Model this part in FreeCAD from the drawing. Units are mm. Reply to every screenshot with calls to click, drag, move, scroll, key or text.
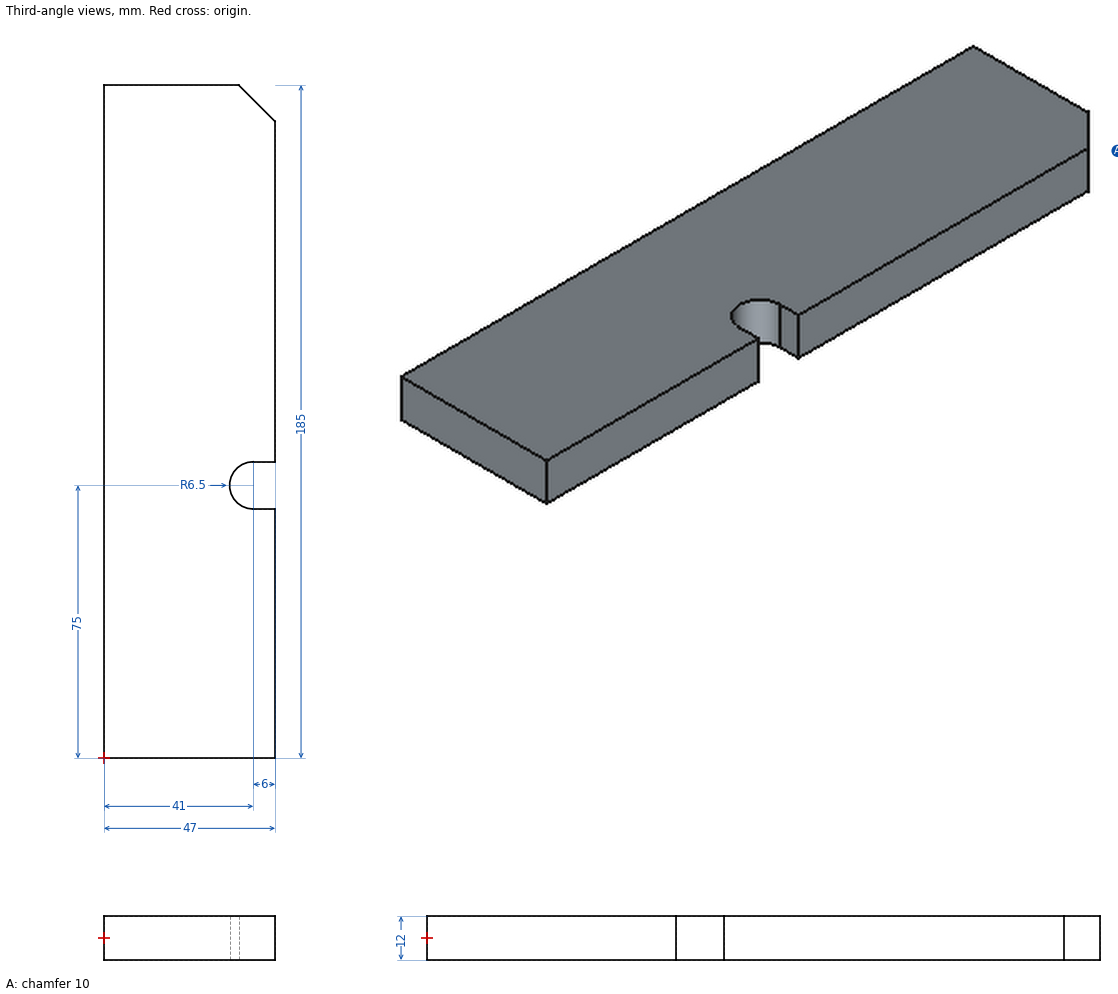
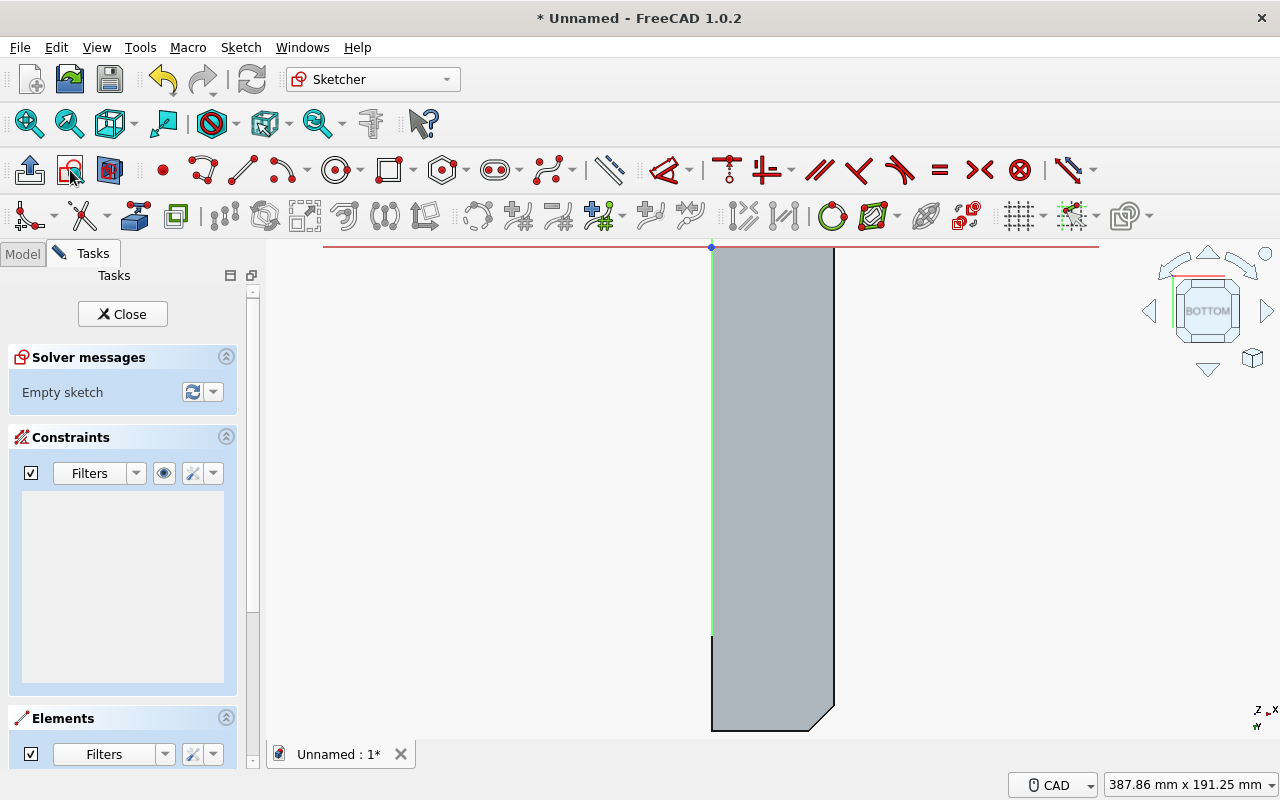
scroll(832, 438, up, 11)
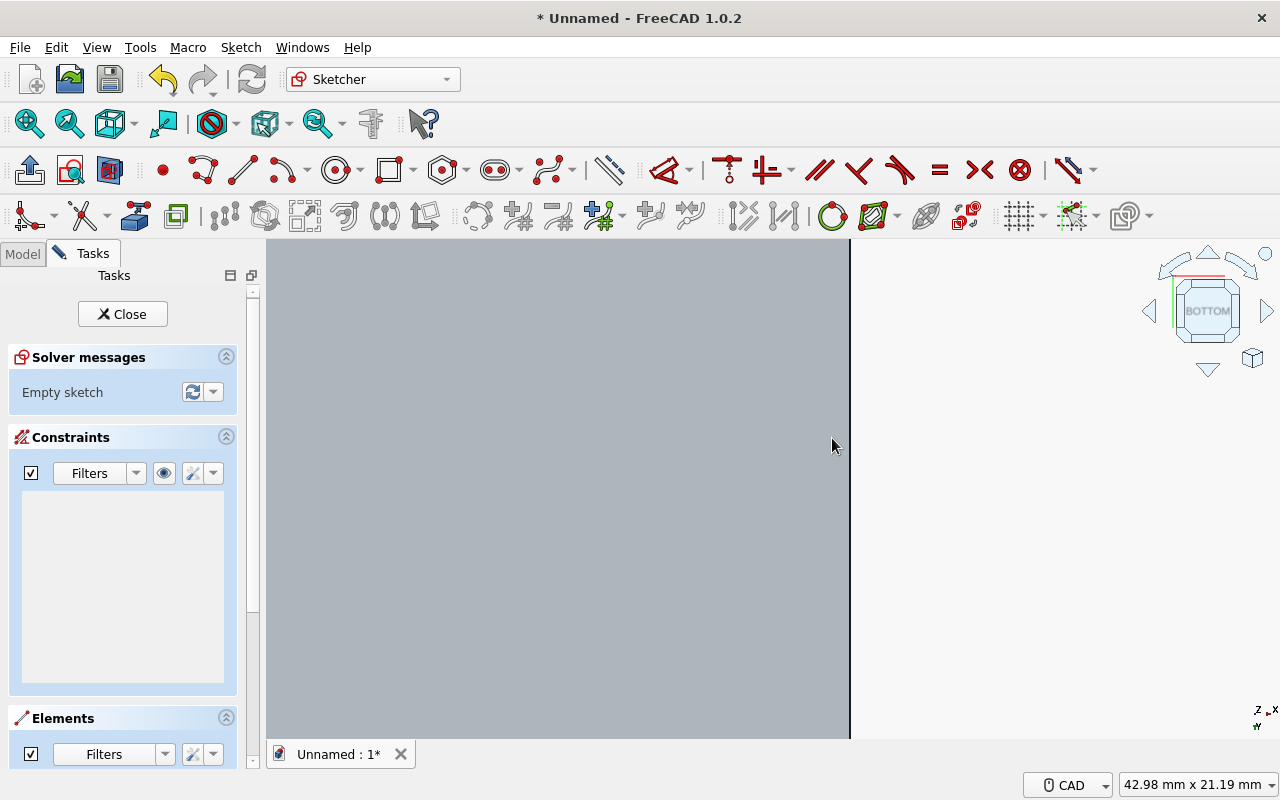
click(204, 170)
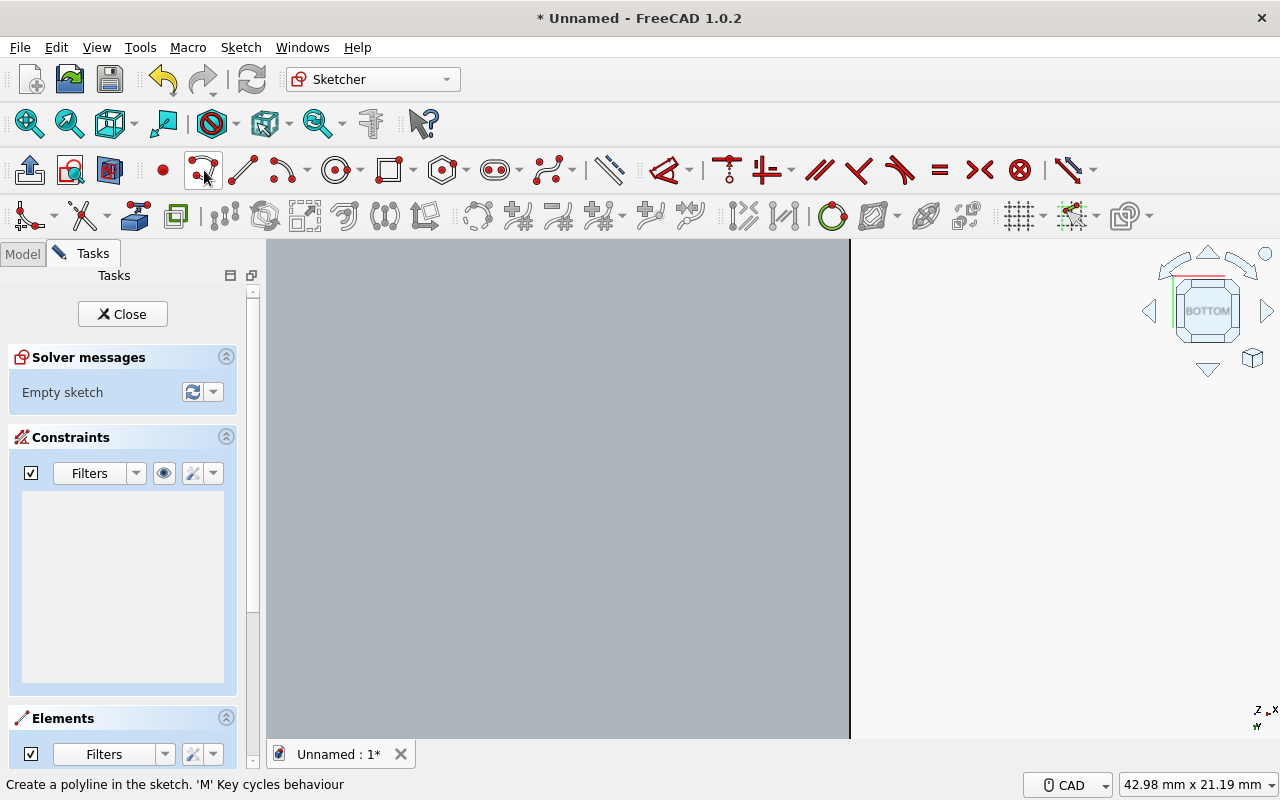
click(708, 636)
click(850, 636)
click(850, 329)
click(708, 329)
right_click(708, 329)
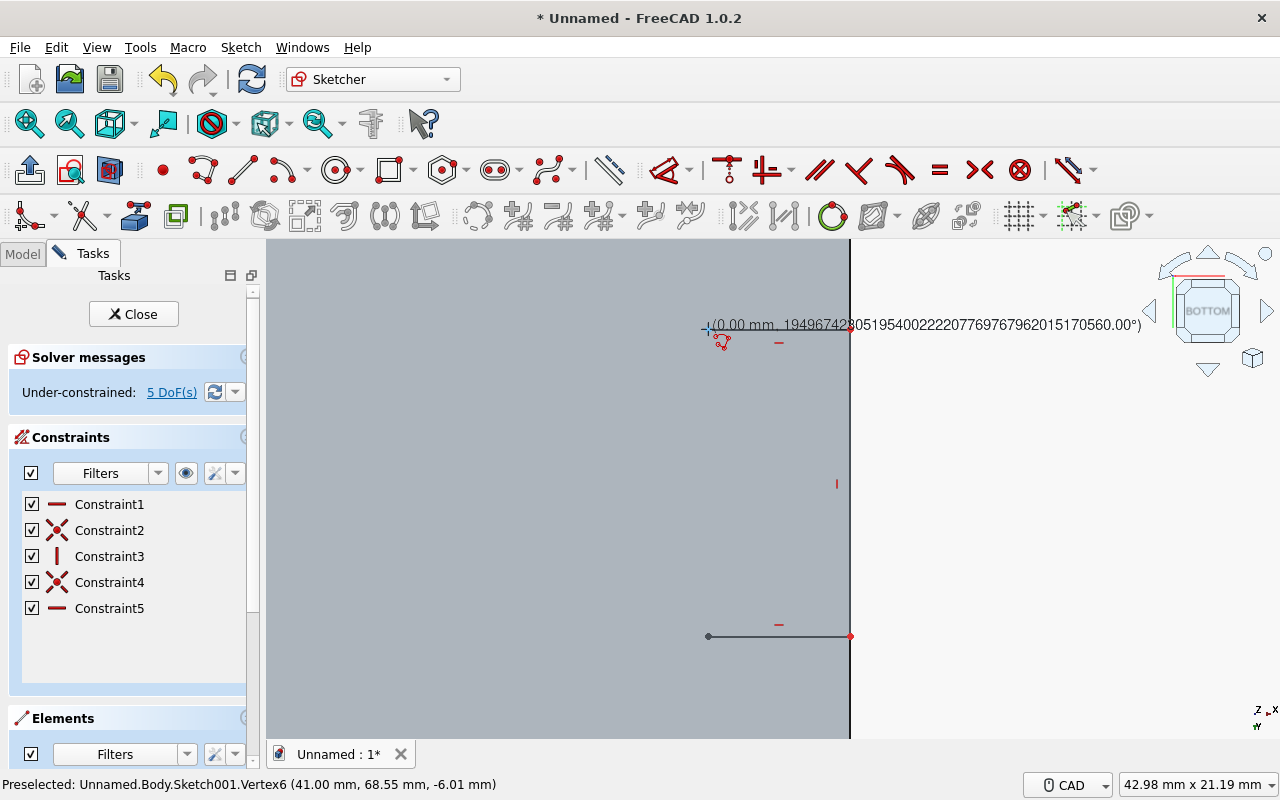
key(g)
key(3)
key(a)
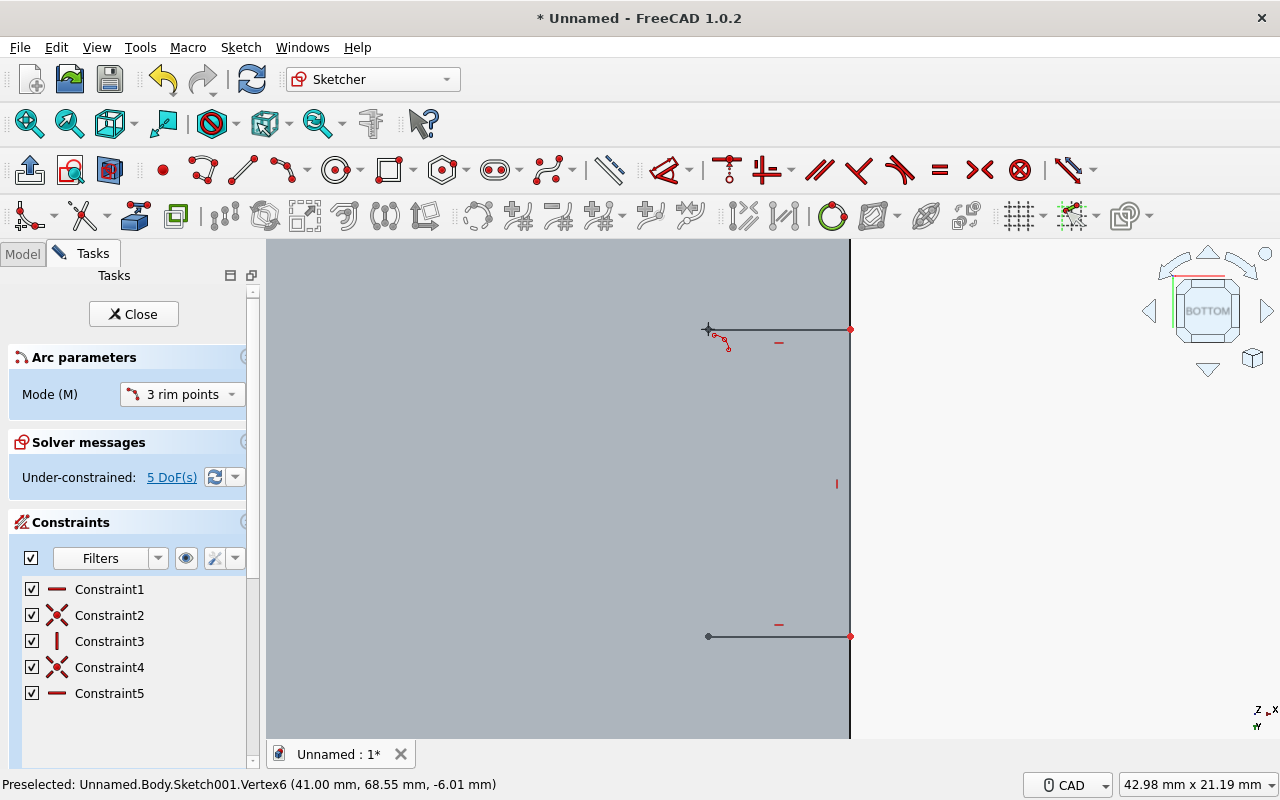
click(708, 330)
click(708, 637)
click(555, 482)
key(Escape)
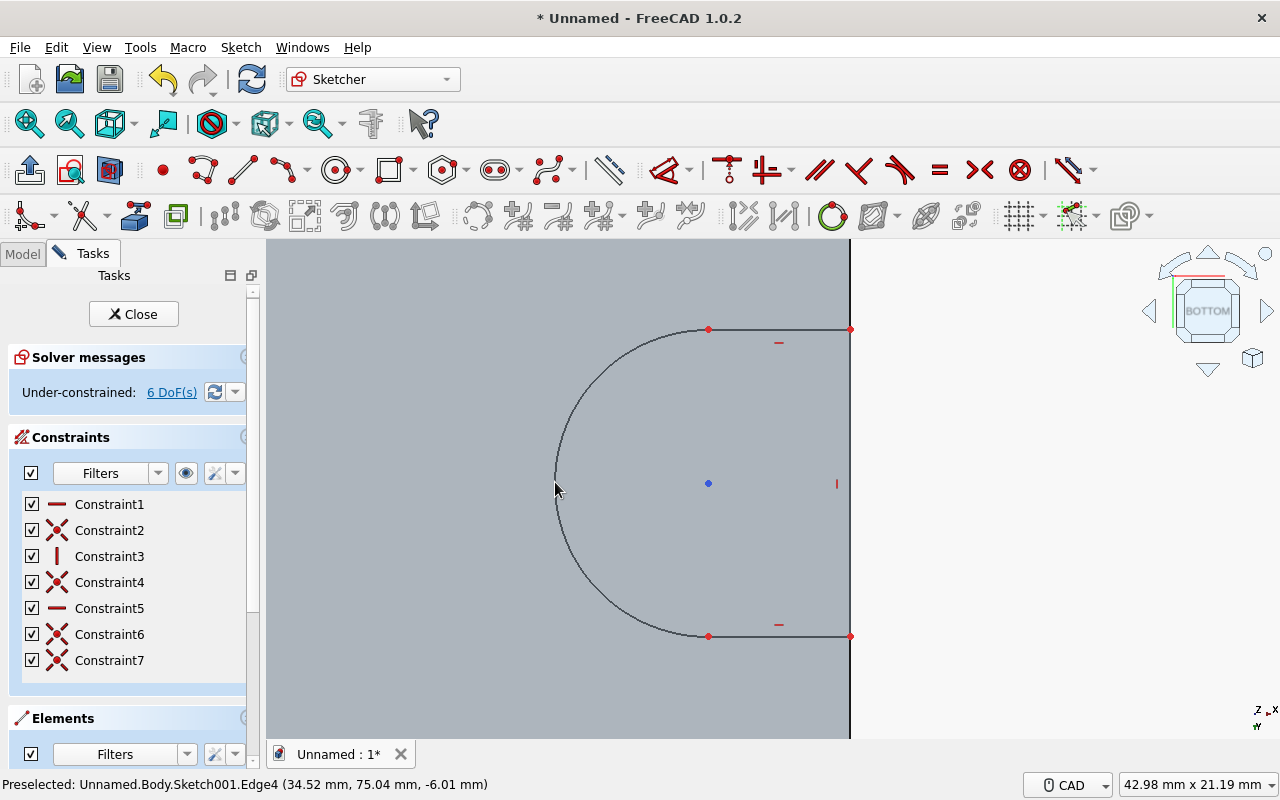
click(751, 637)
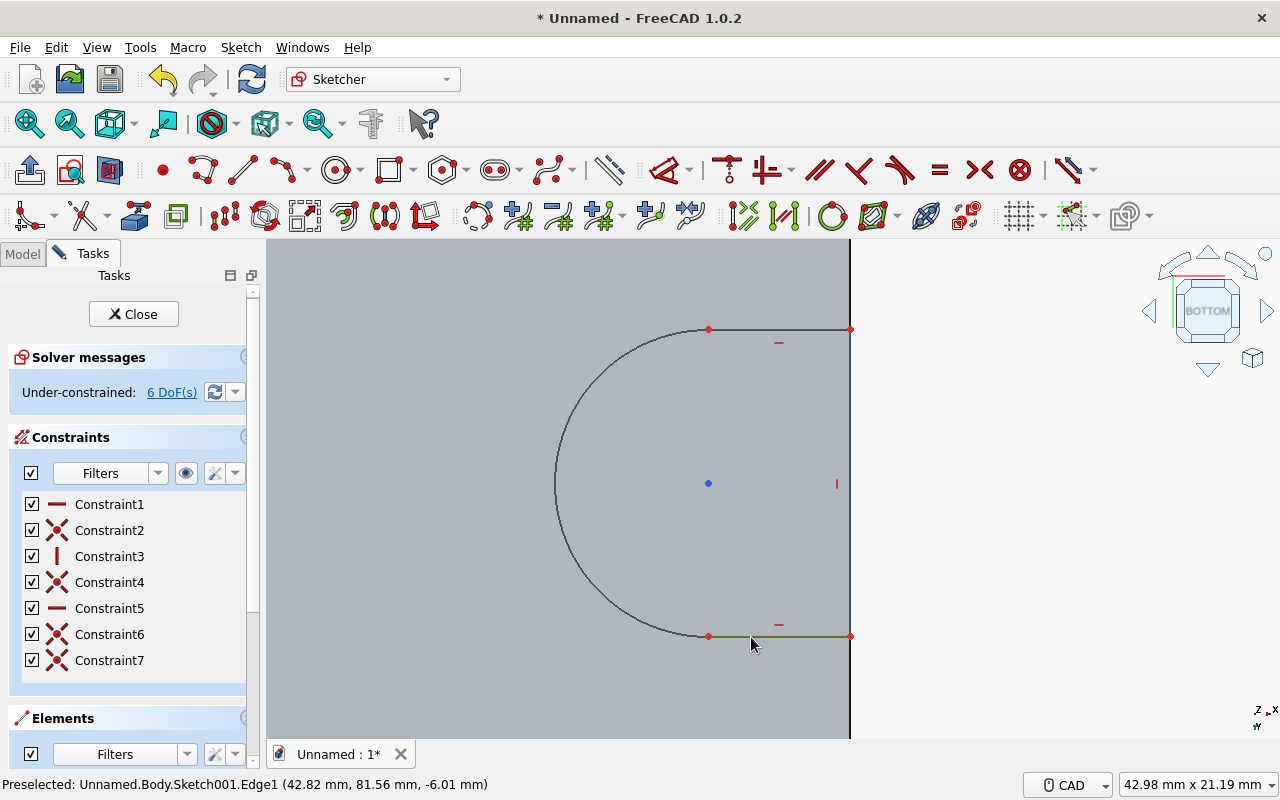
click(584, 393)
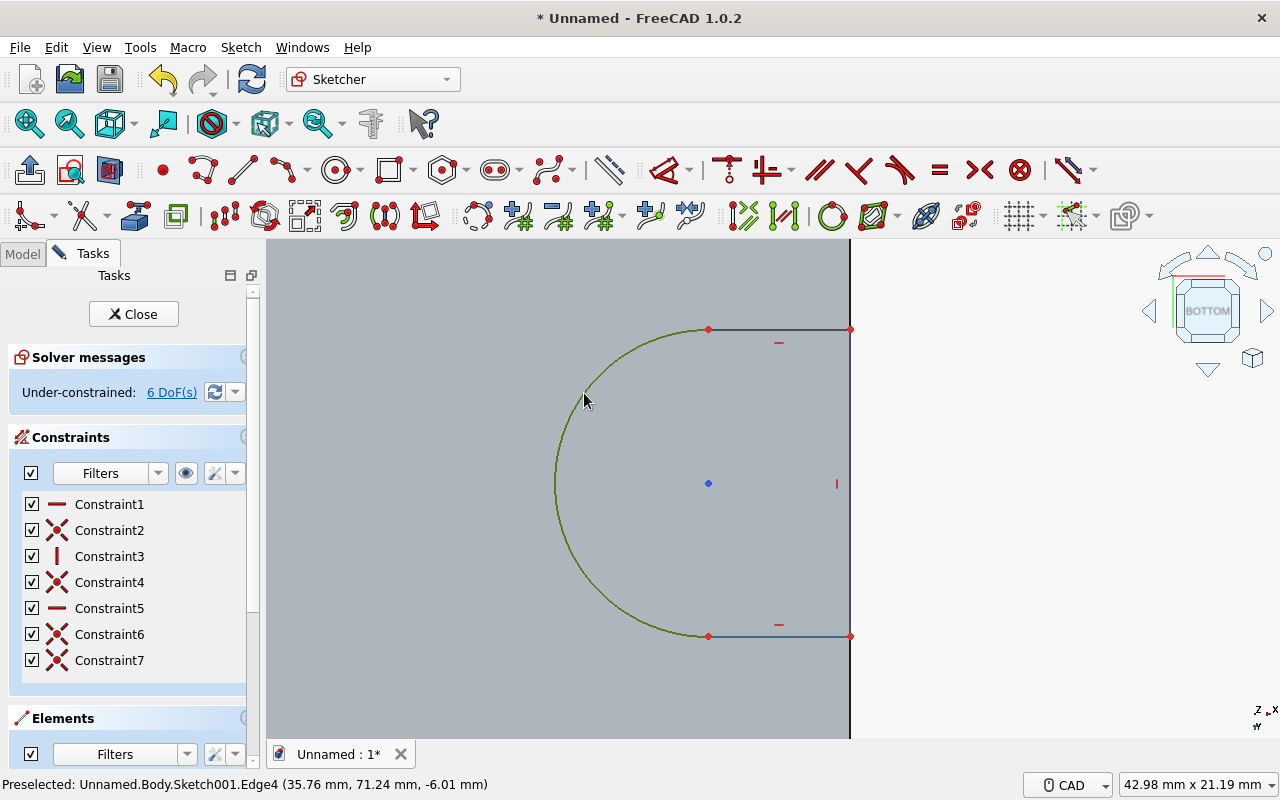
click(900, 170)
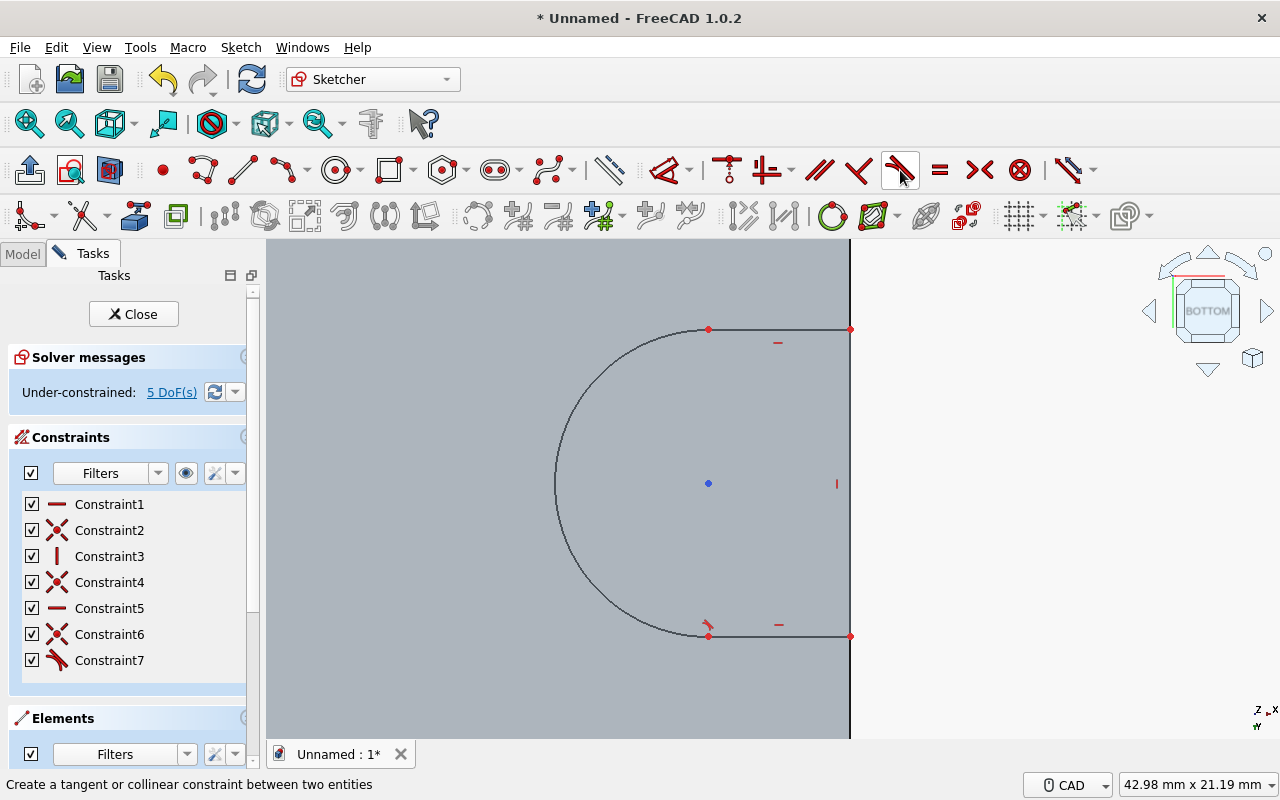
click(807, 330)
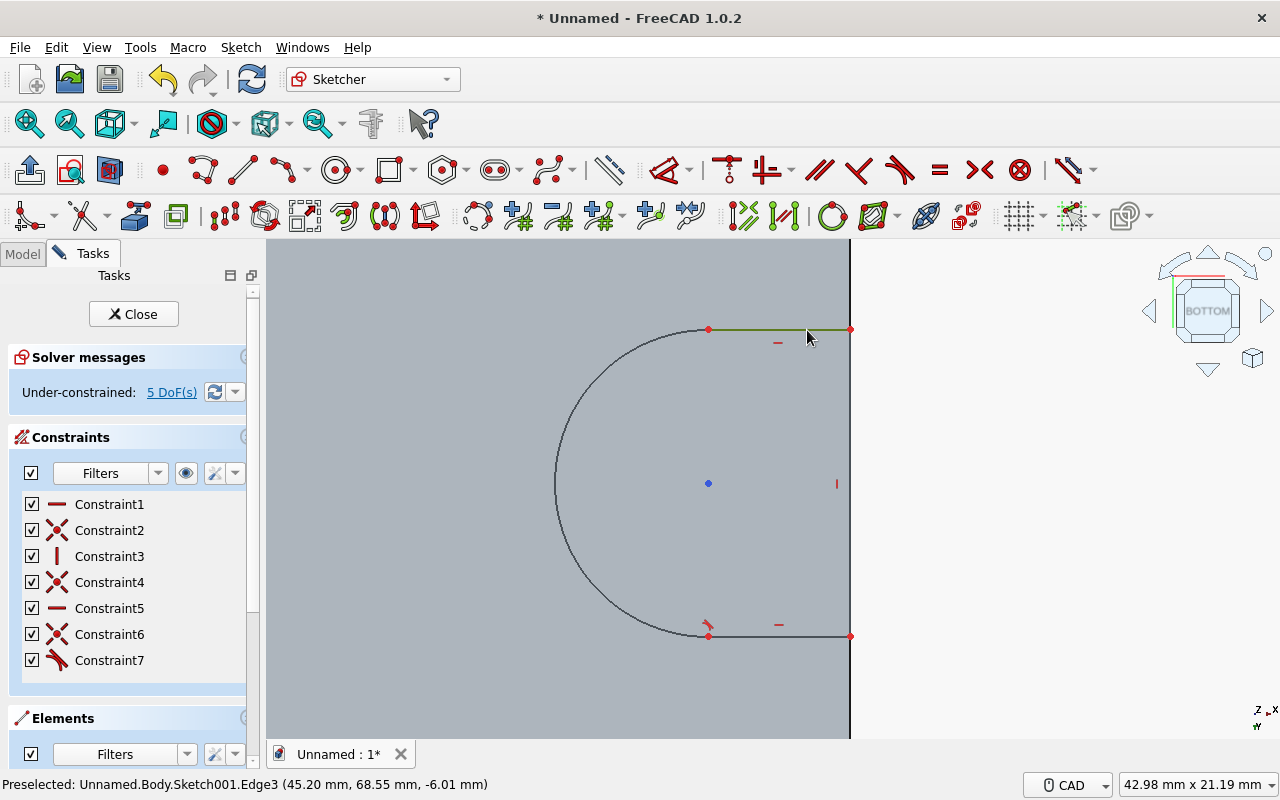
click(584, 394)